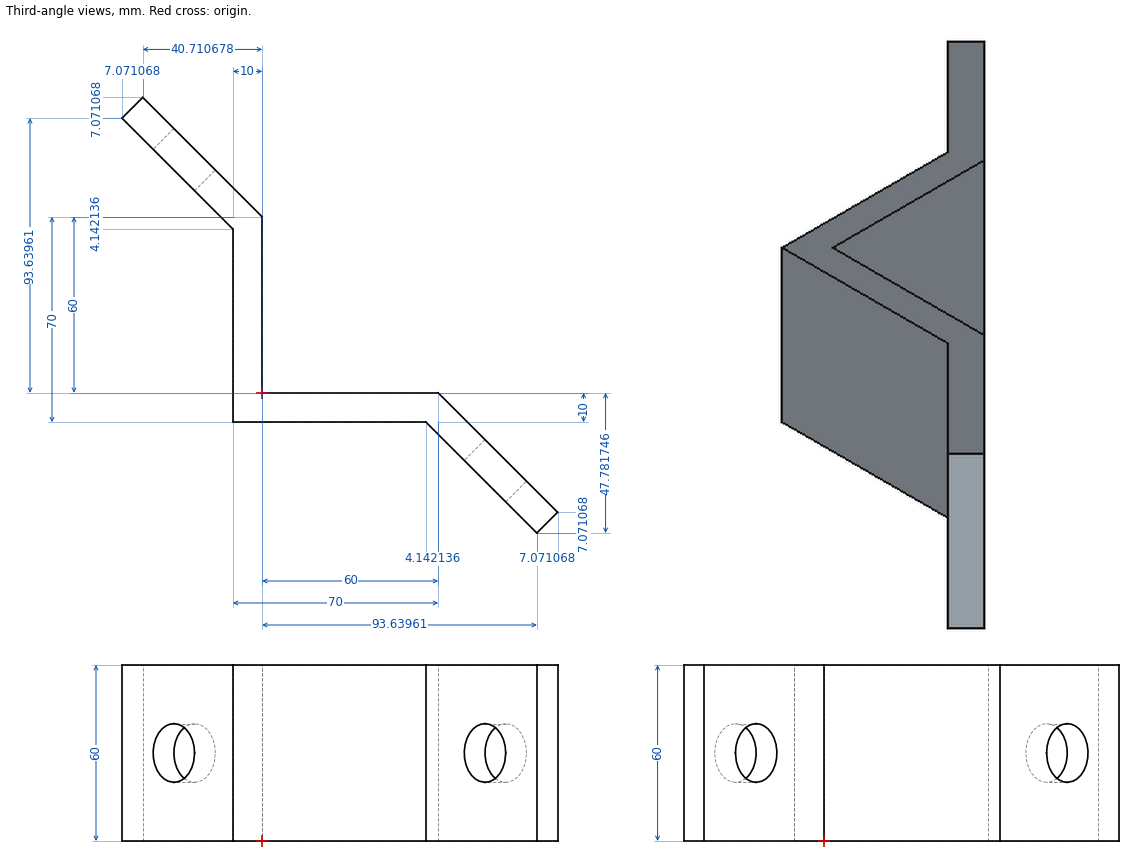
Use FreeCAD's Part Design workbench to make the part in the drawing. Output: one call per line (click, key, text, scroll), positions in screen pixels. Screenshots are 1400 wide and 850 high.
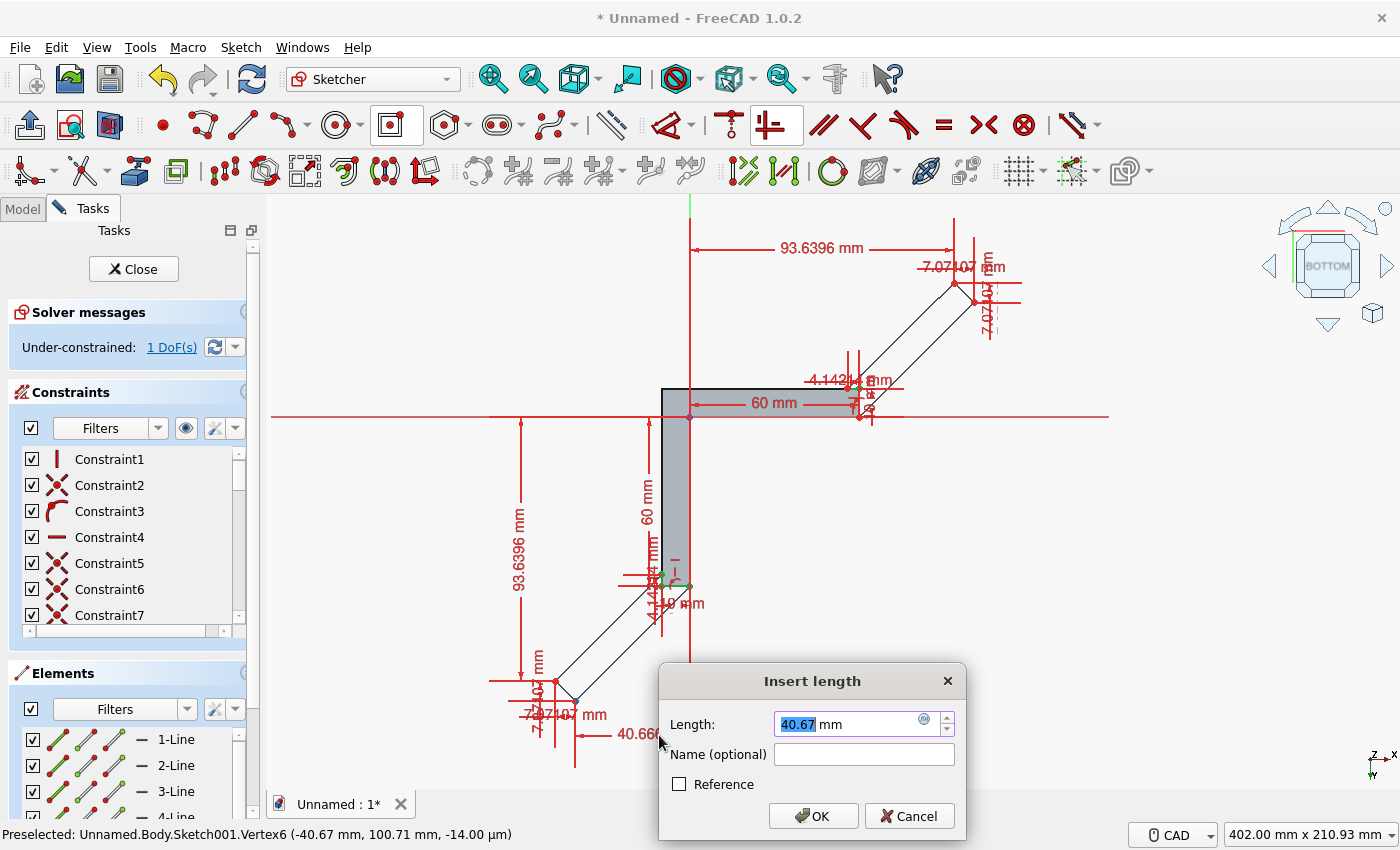
text(40.710678)
key(Return)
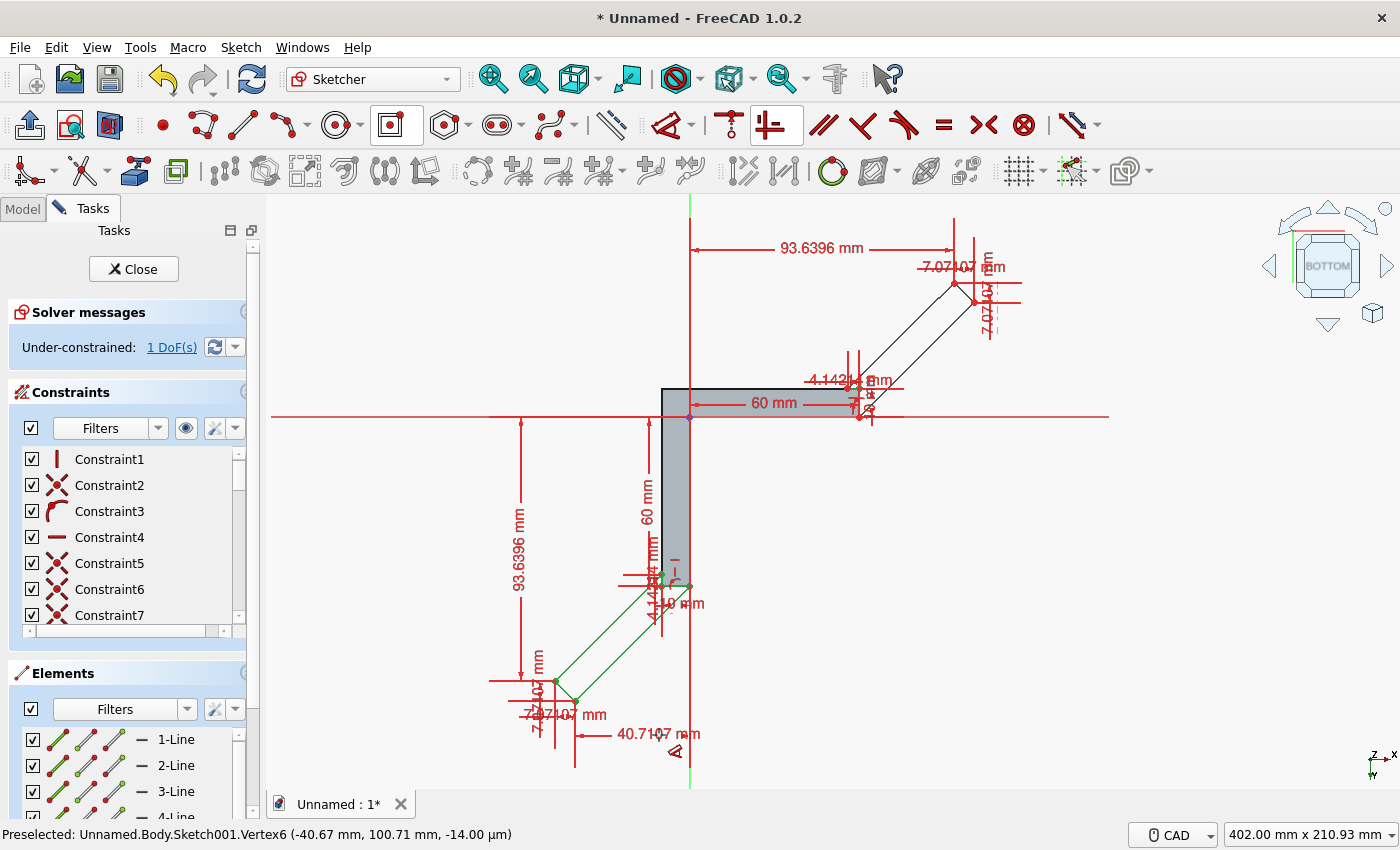
click(954, 283)
click(988, 350)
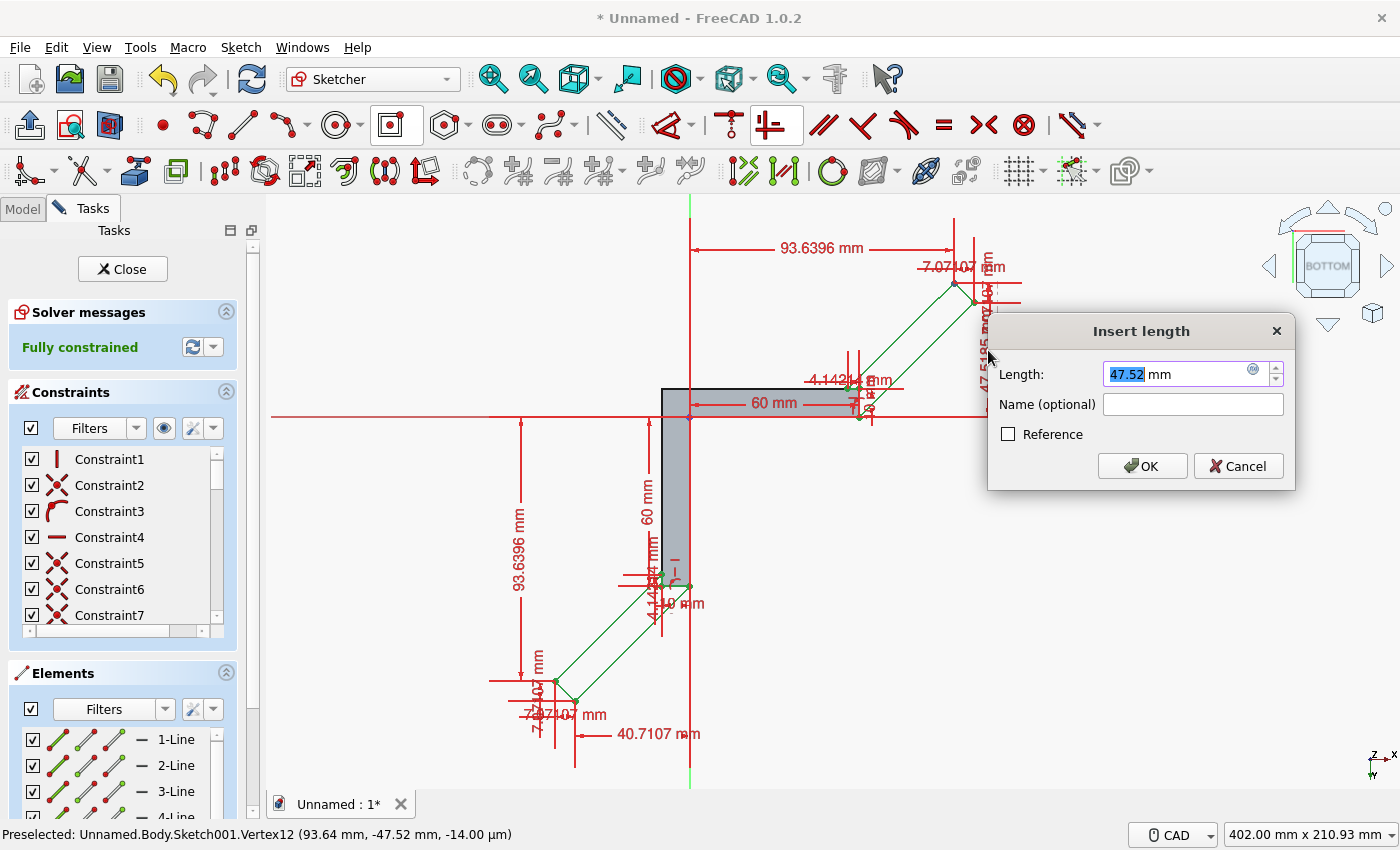
text(47.781746)
key(Return)
key(Escape)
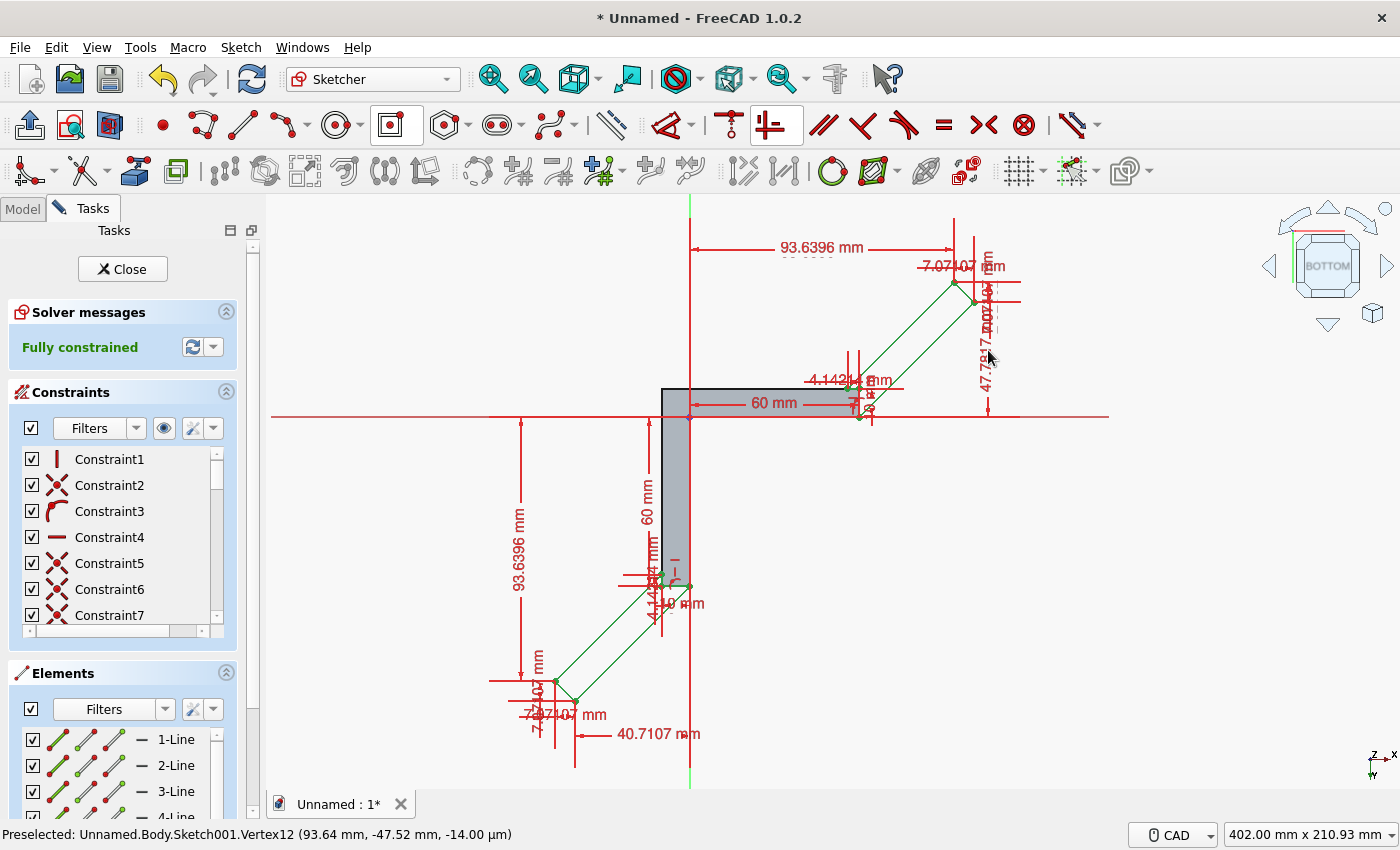
click(123, 269)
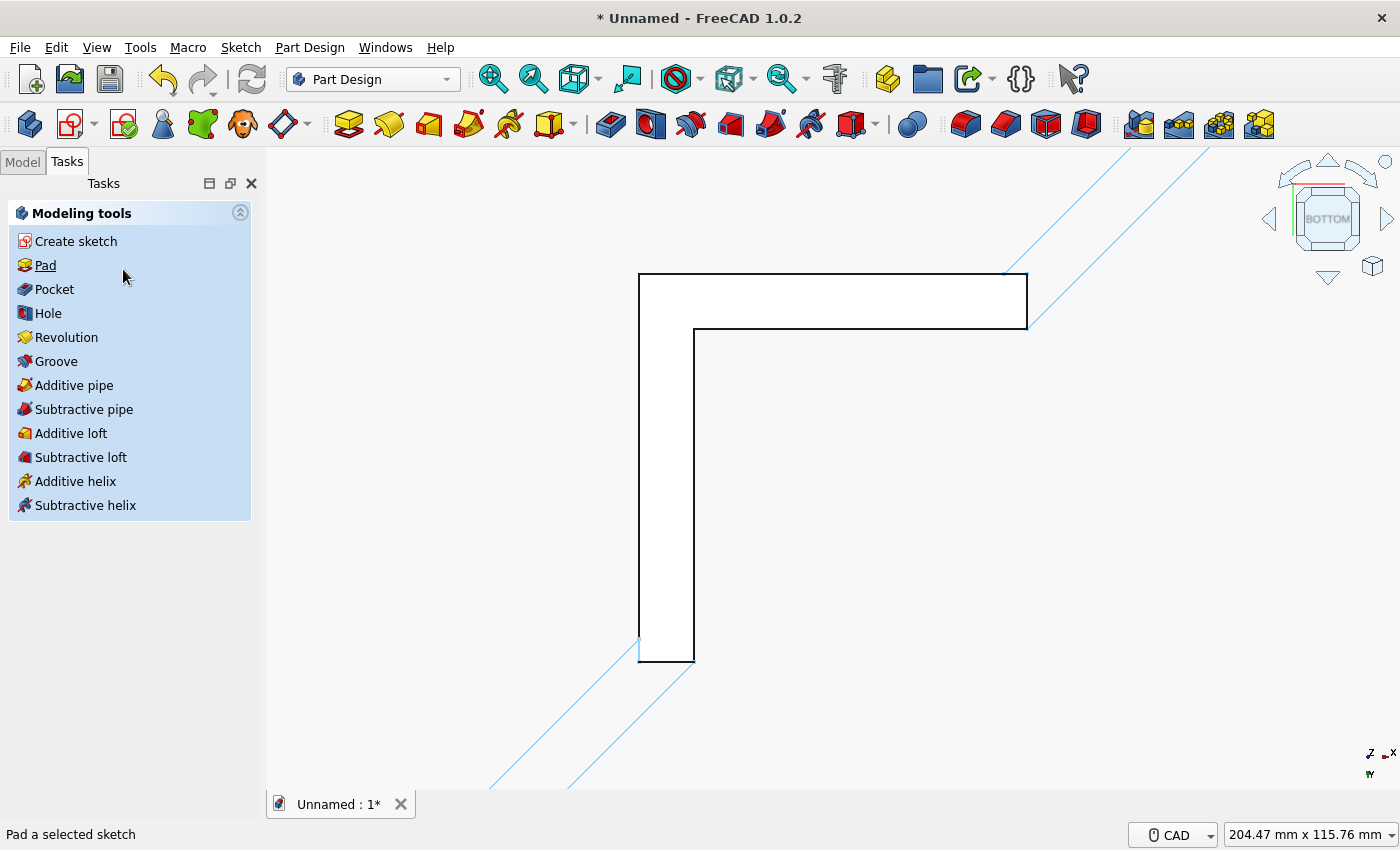
click(350, 124)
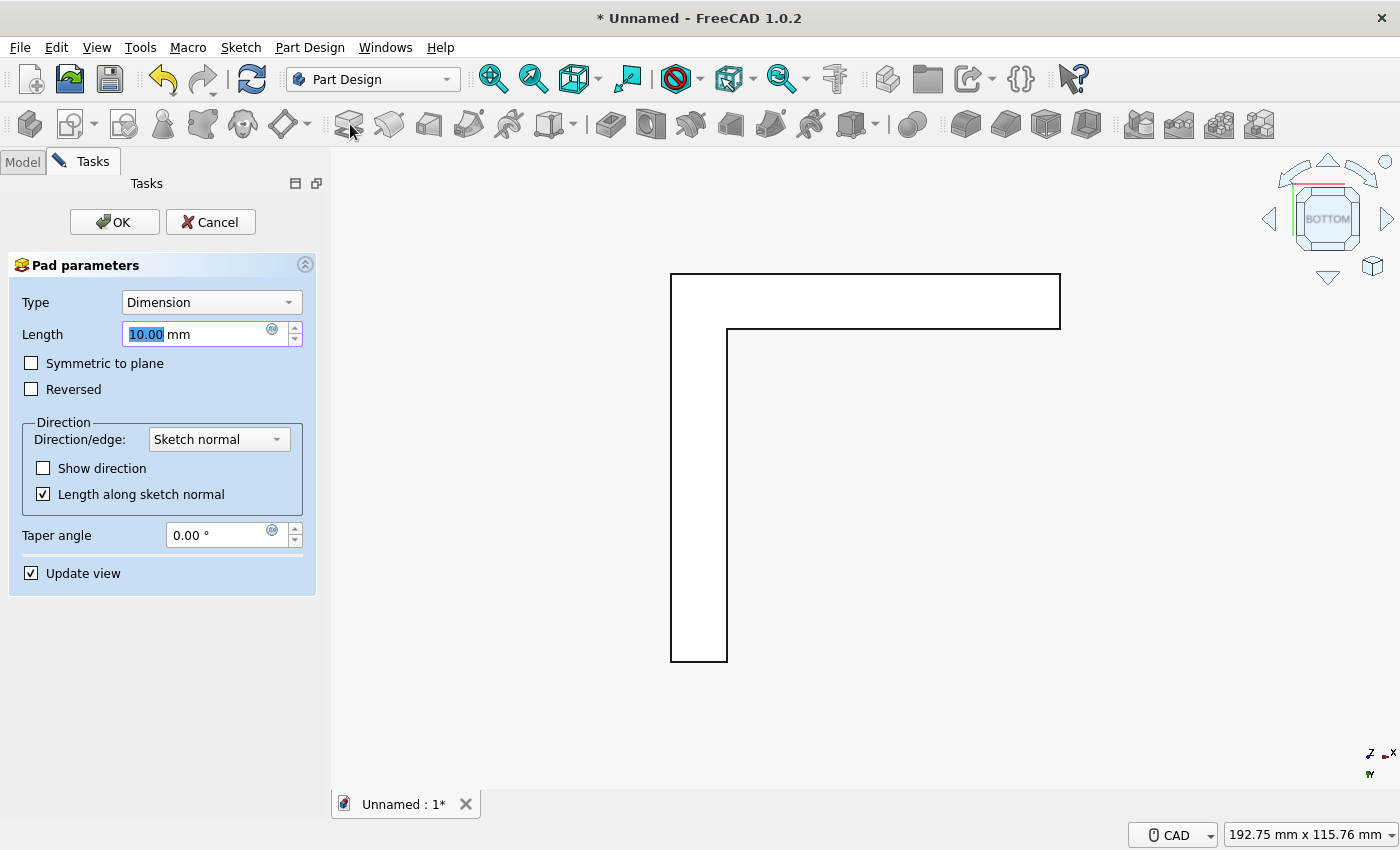
text(60)
key(Tab)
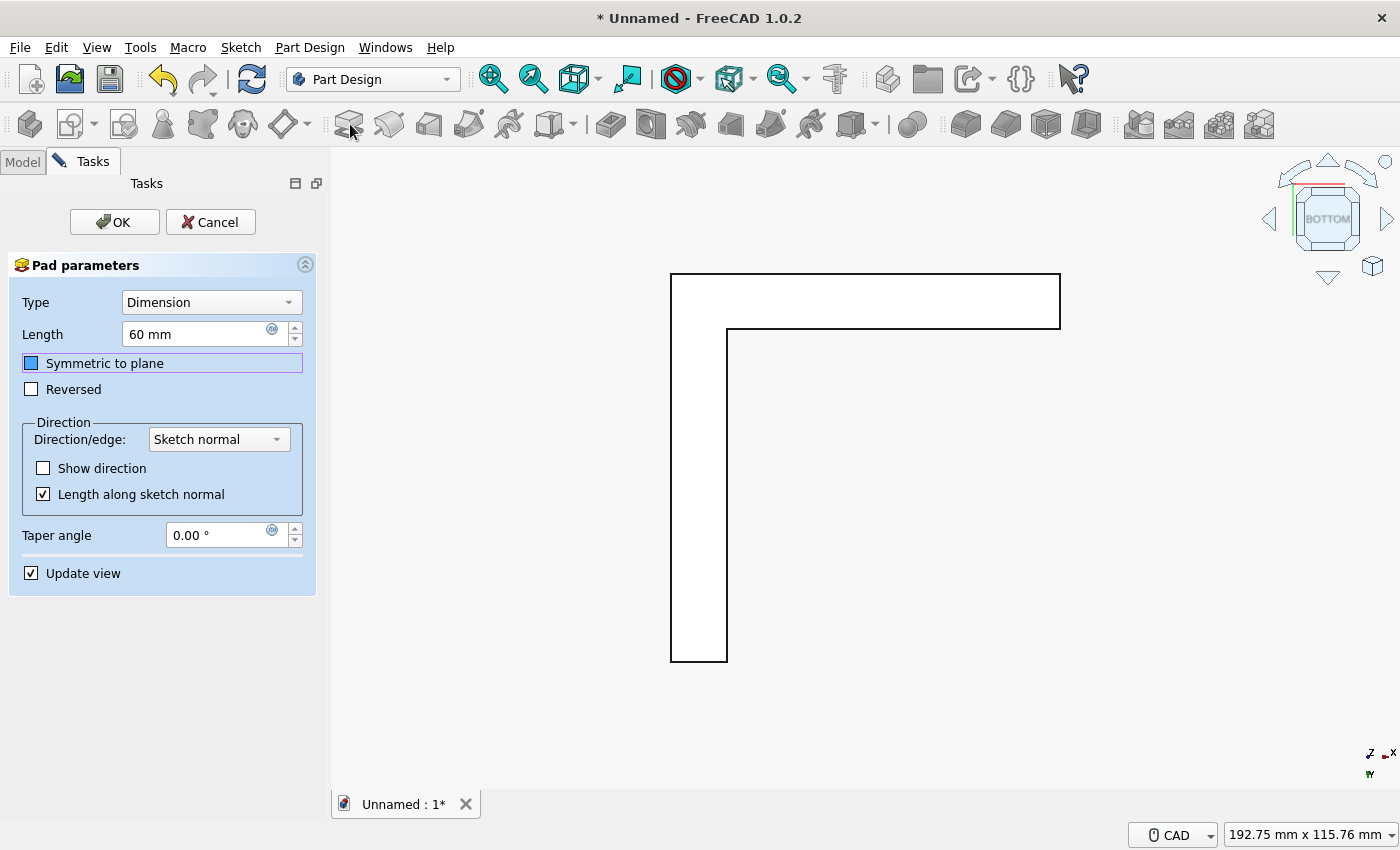
click(30, 389)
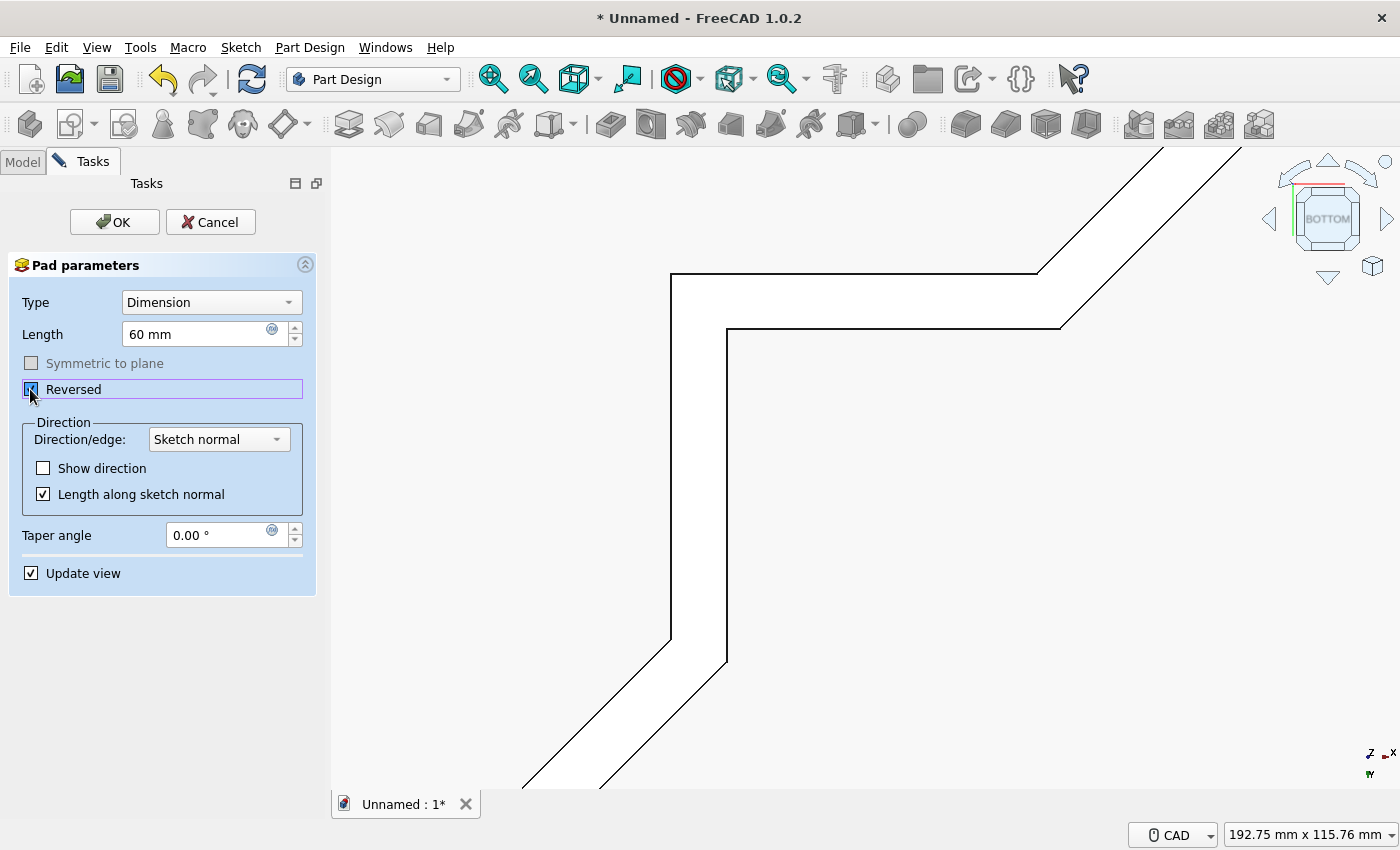
click(115, 222)